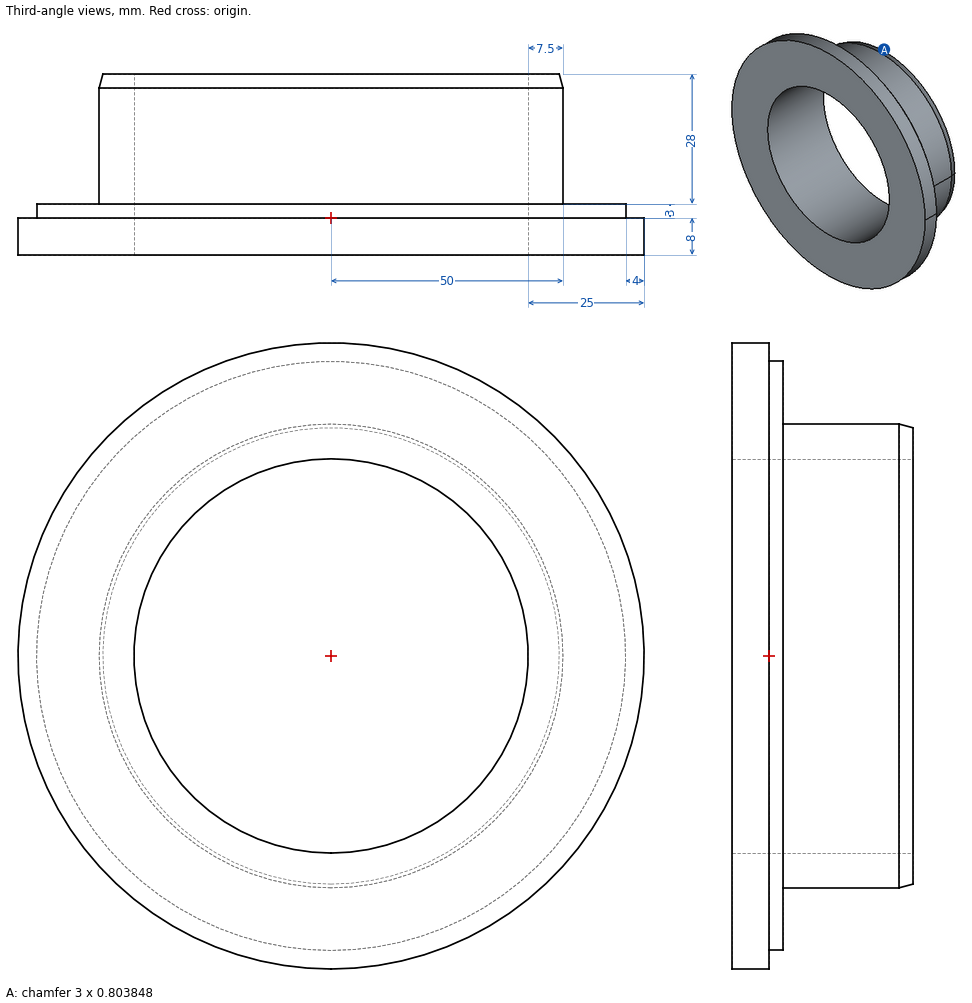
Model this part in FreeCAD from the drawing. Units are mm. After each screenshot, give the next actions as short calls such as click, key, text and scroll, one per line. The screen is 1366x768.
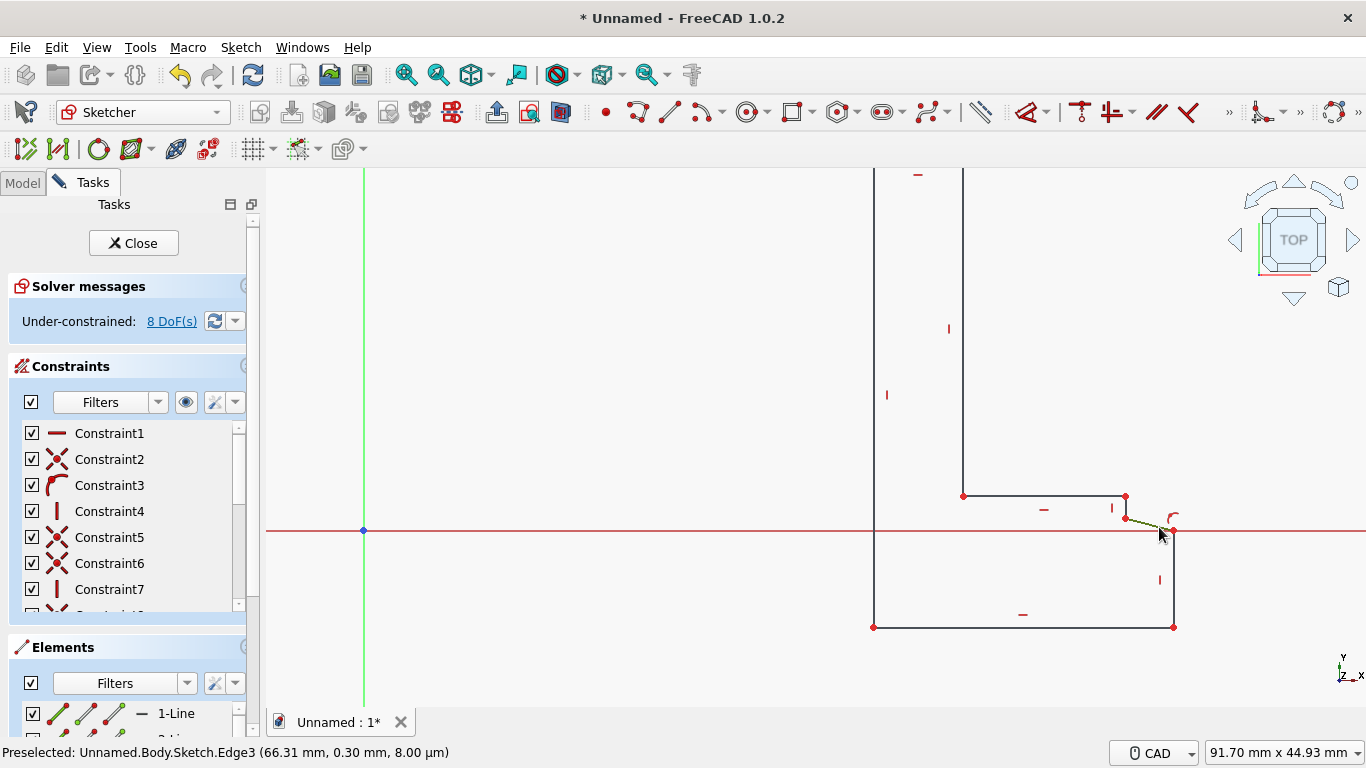
click(1134, 112)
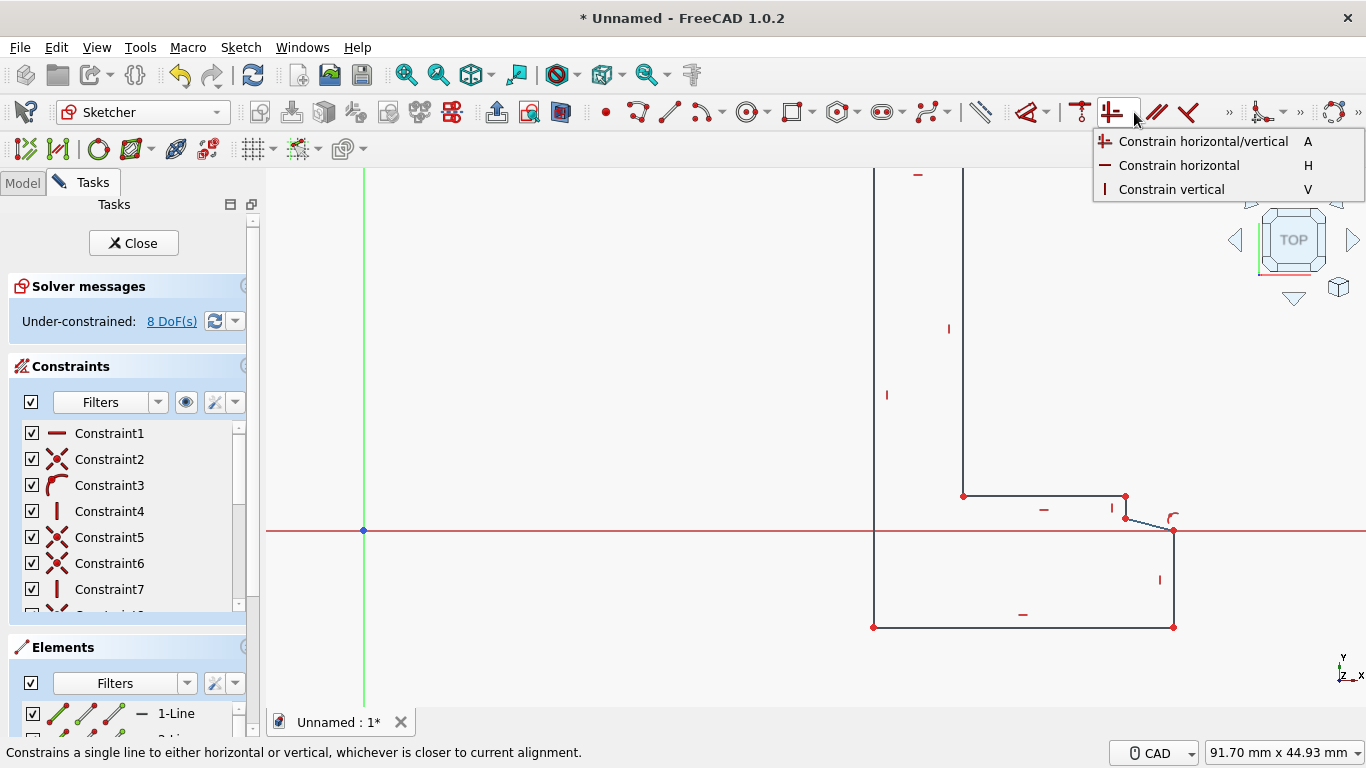
click(1229, 165)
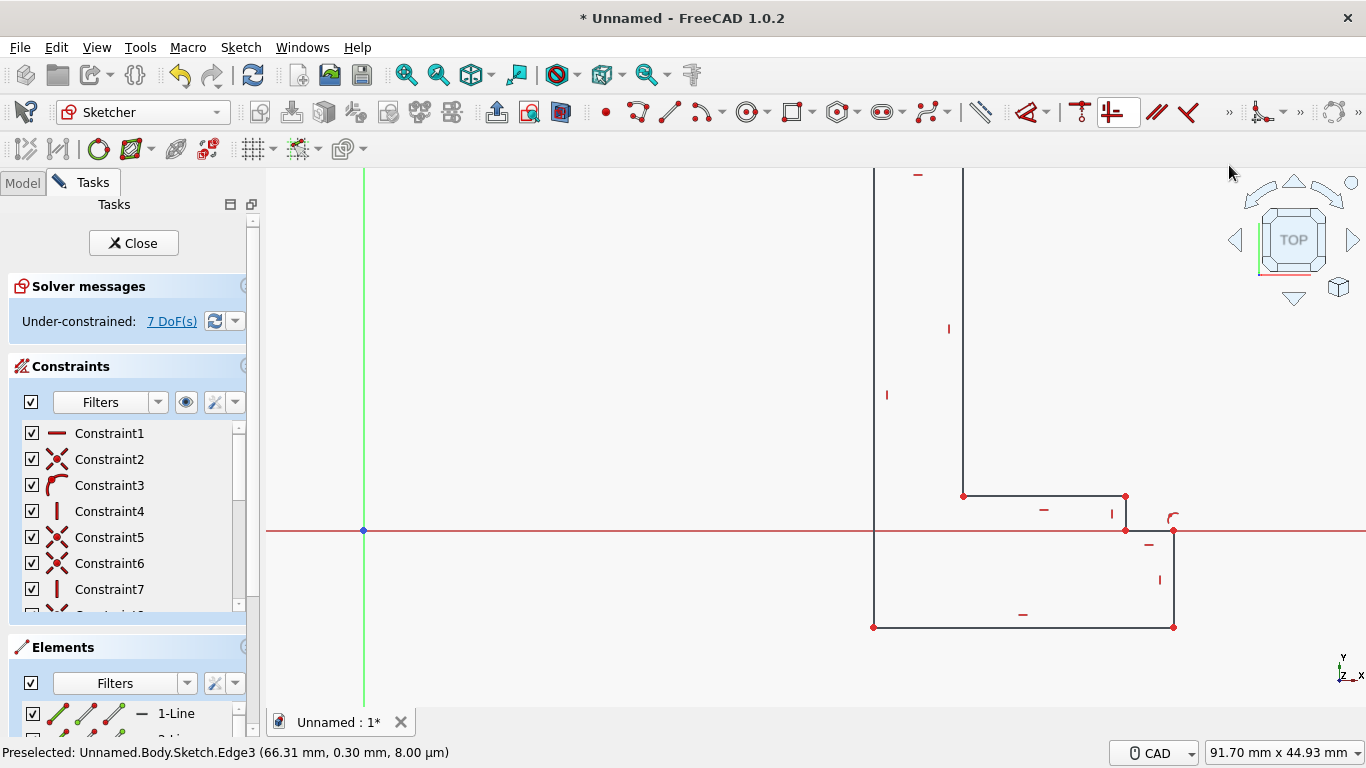
click(1026, 112)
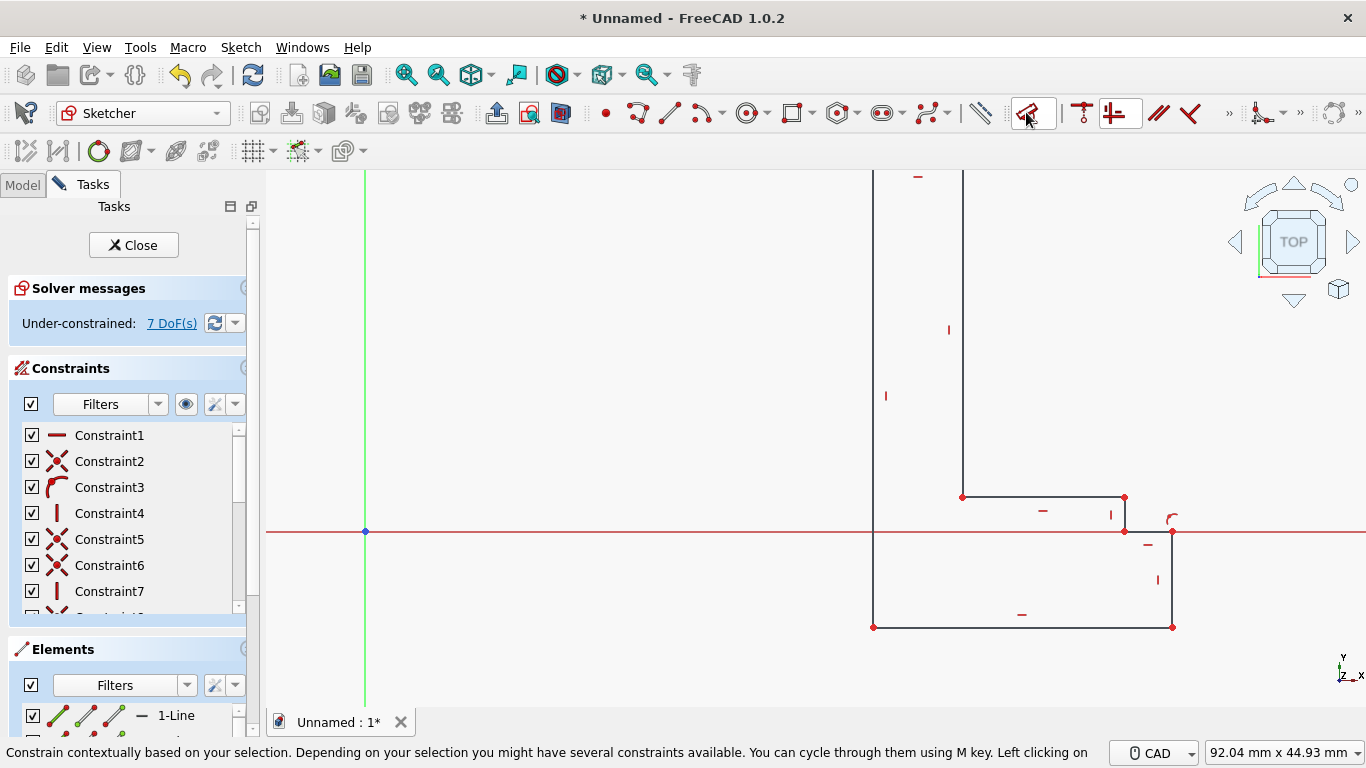
click(1172, 599)
click(1138, 580)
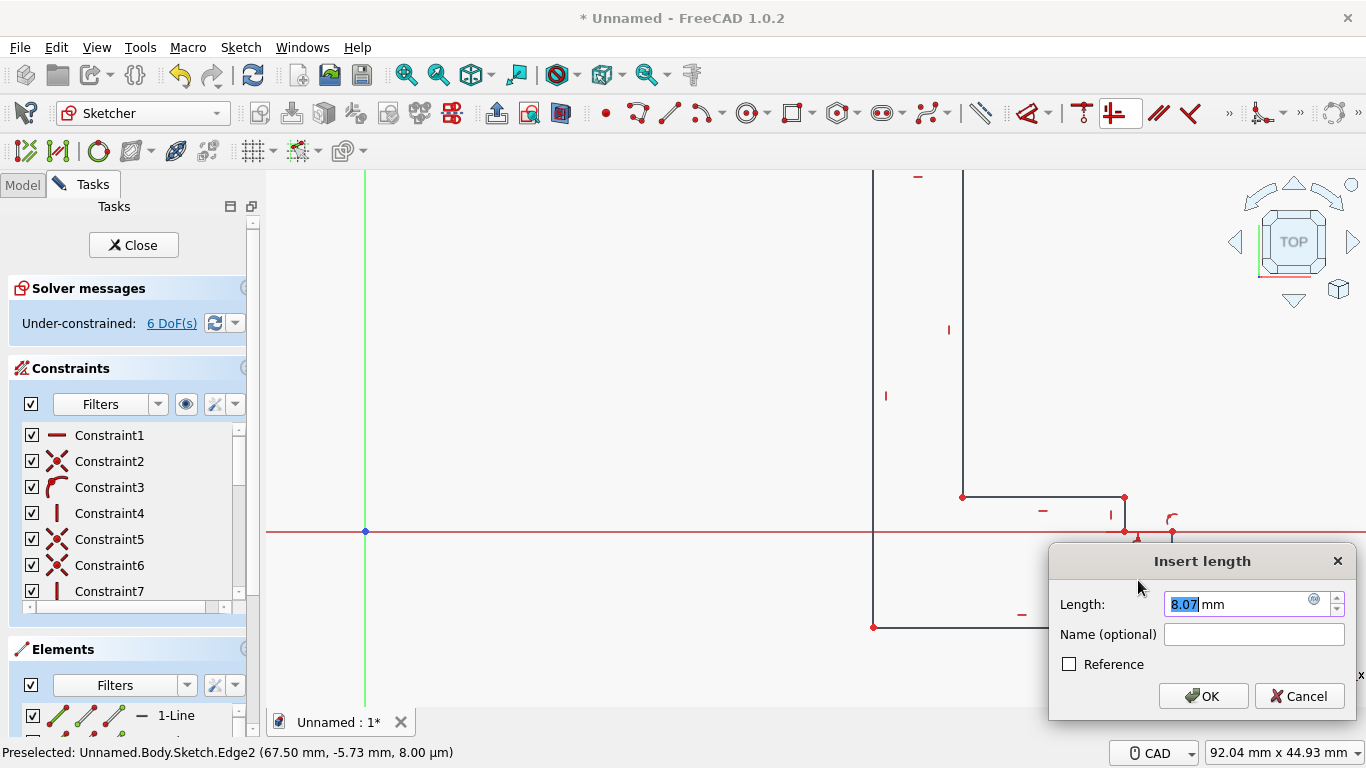
text(8)
key(Return)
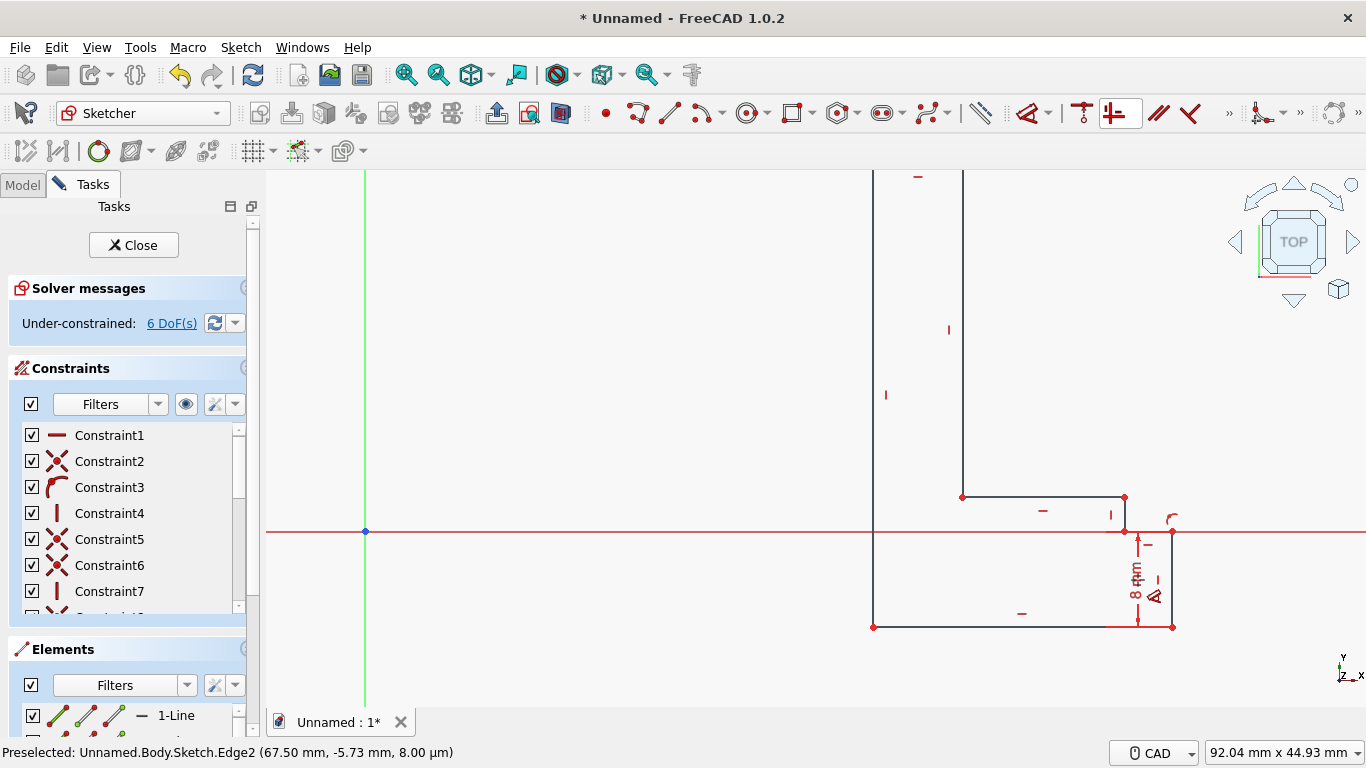
click(1158, 532)
click(1148, 498)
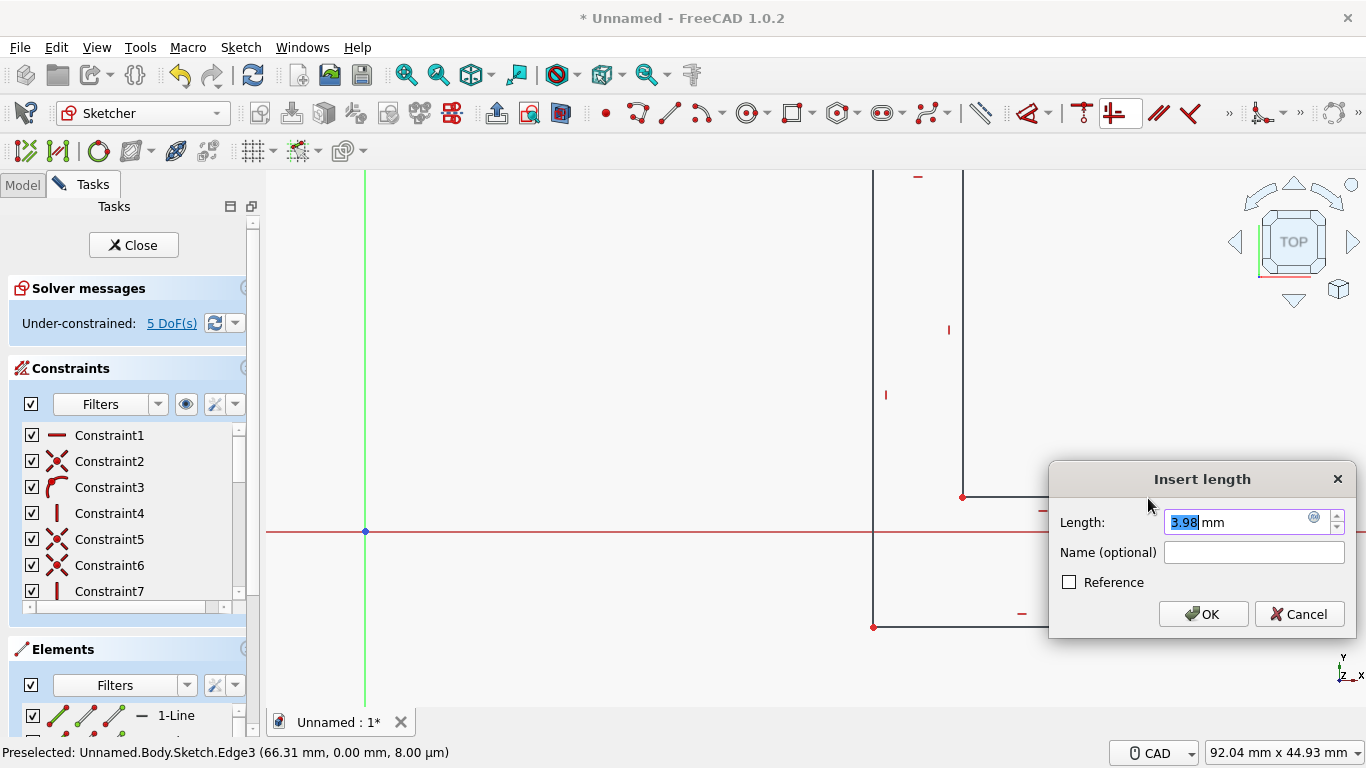
text(4)
key(Return)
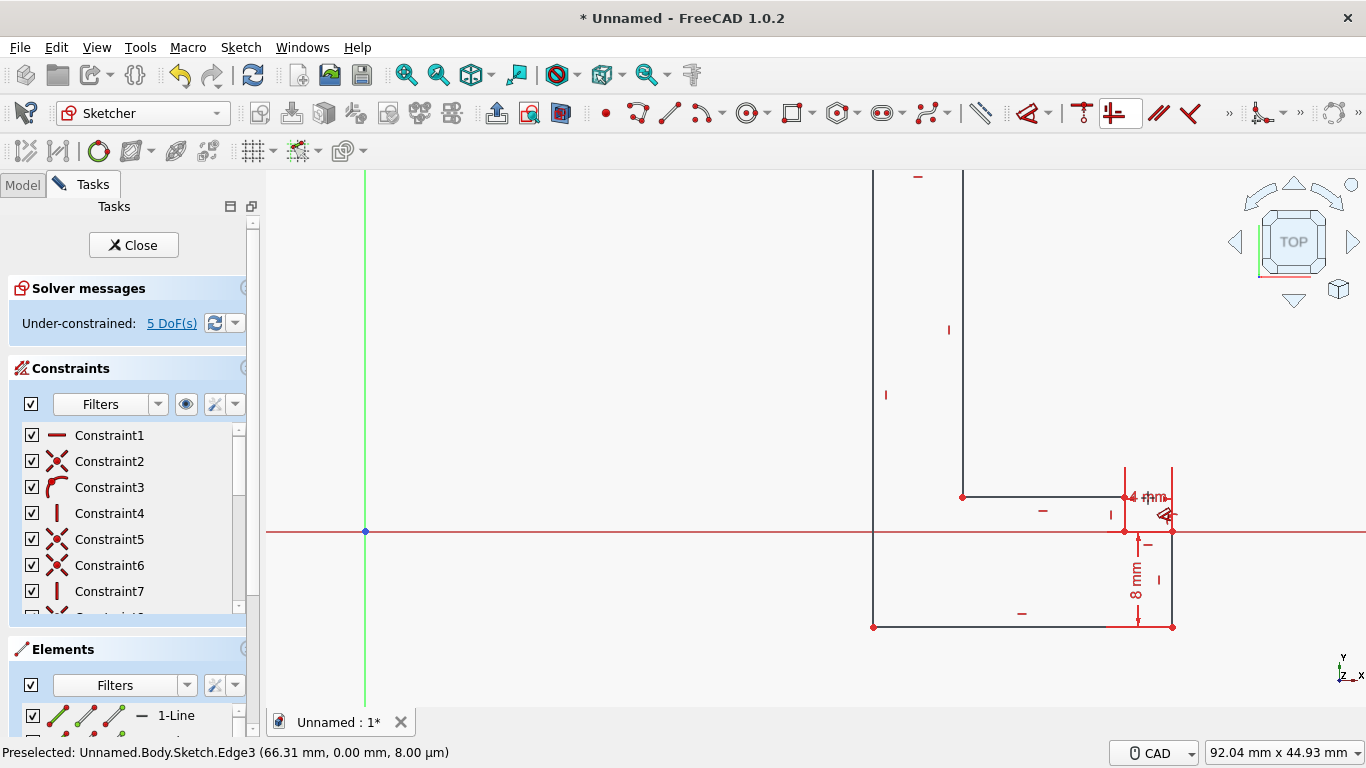
scroll(1125, 521, up, 2)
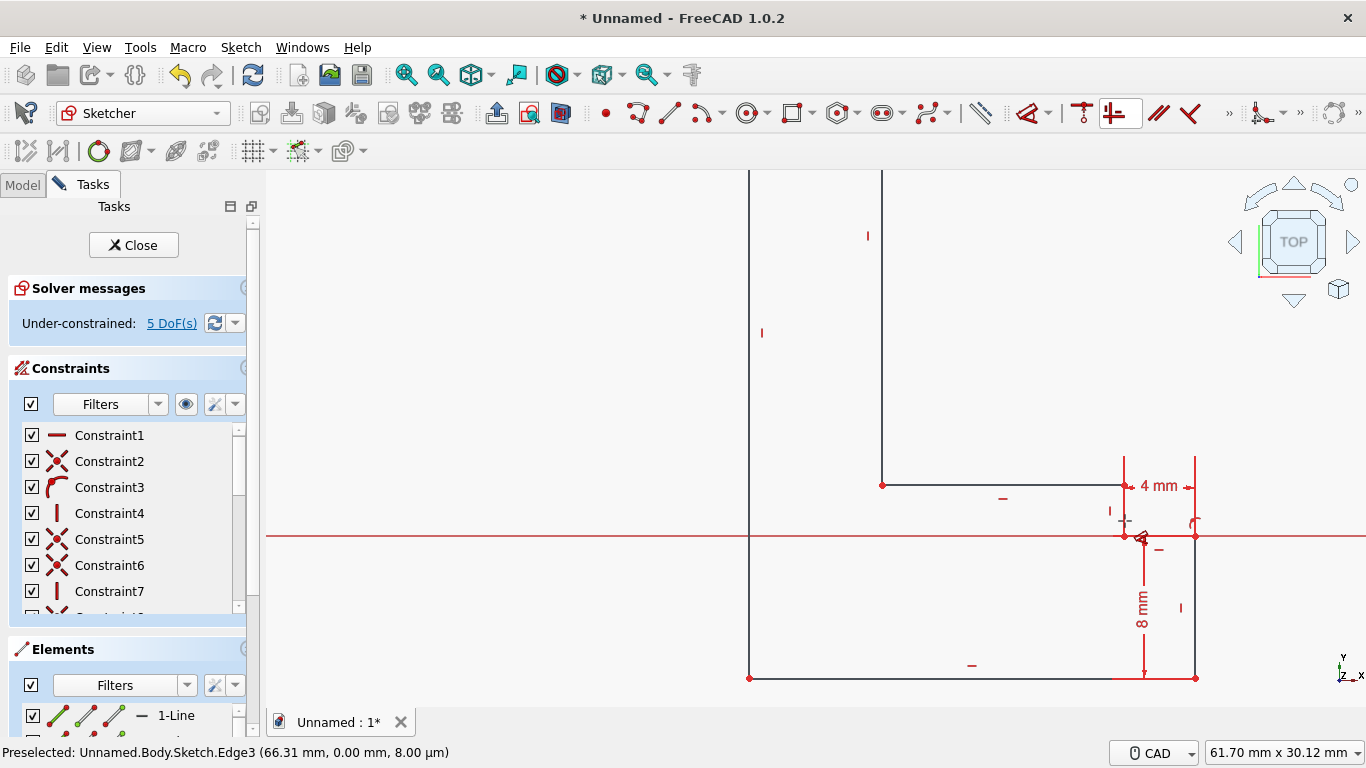
click(1124, 521)
click(1158, 511)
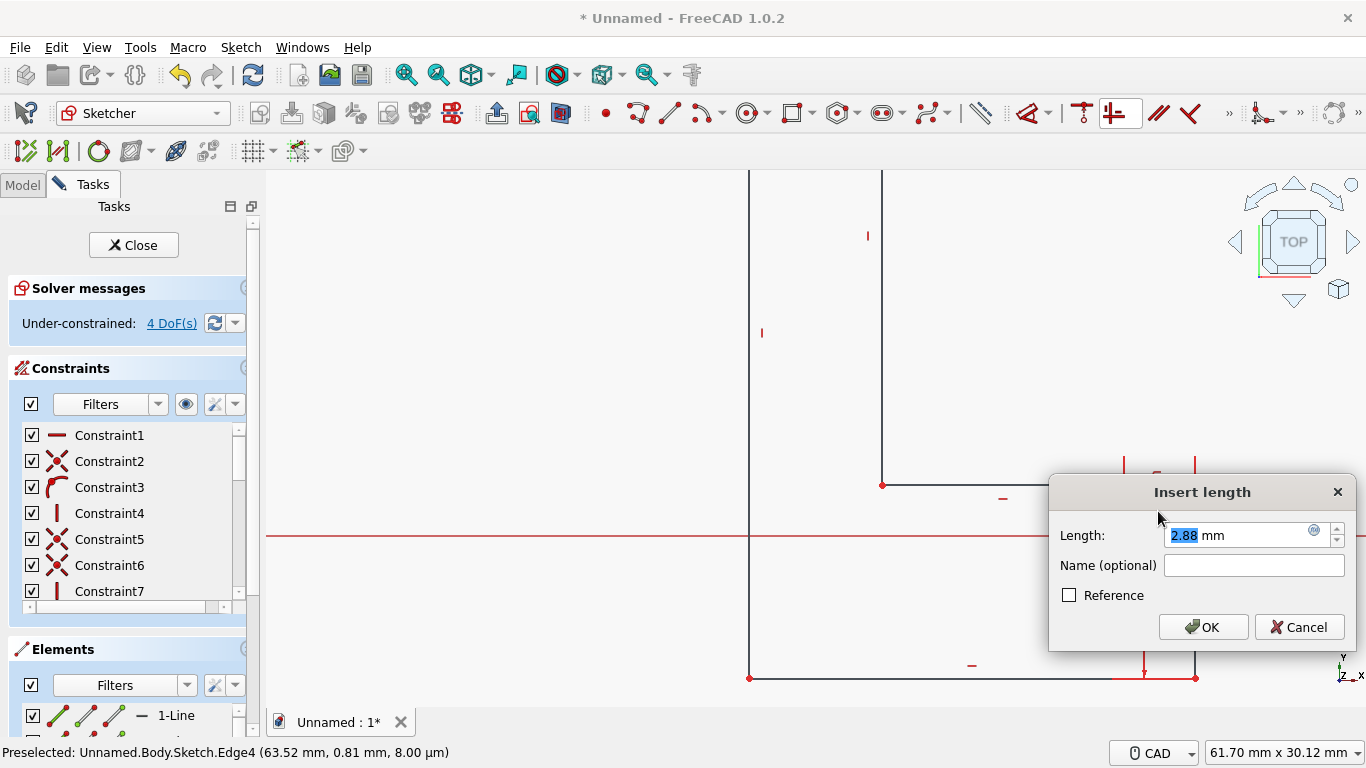
text(3)
key(Return)